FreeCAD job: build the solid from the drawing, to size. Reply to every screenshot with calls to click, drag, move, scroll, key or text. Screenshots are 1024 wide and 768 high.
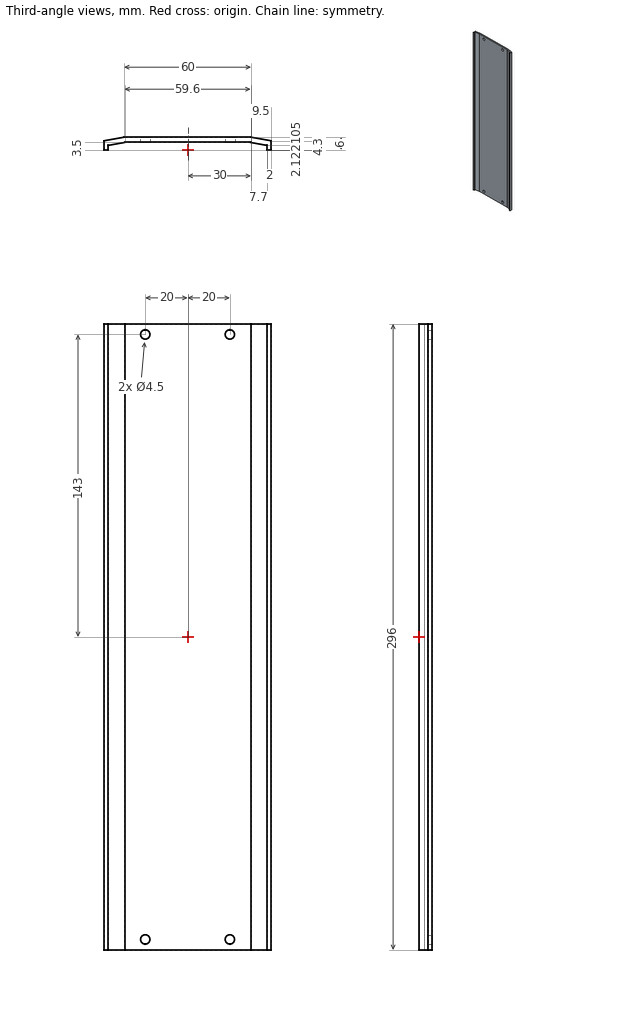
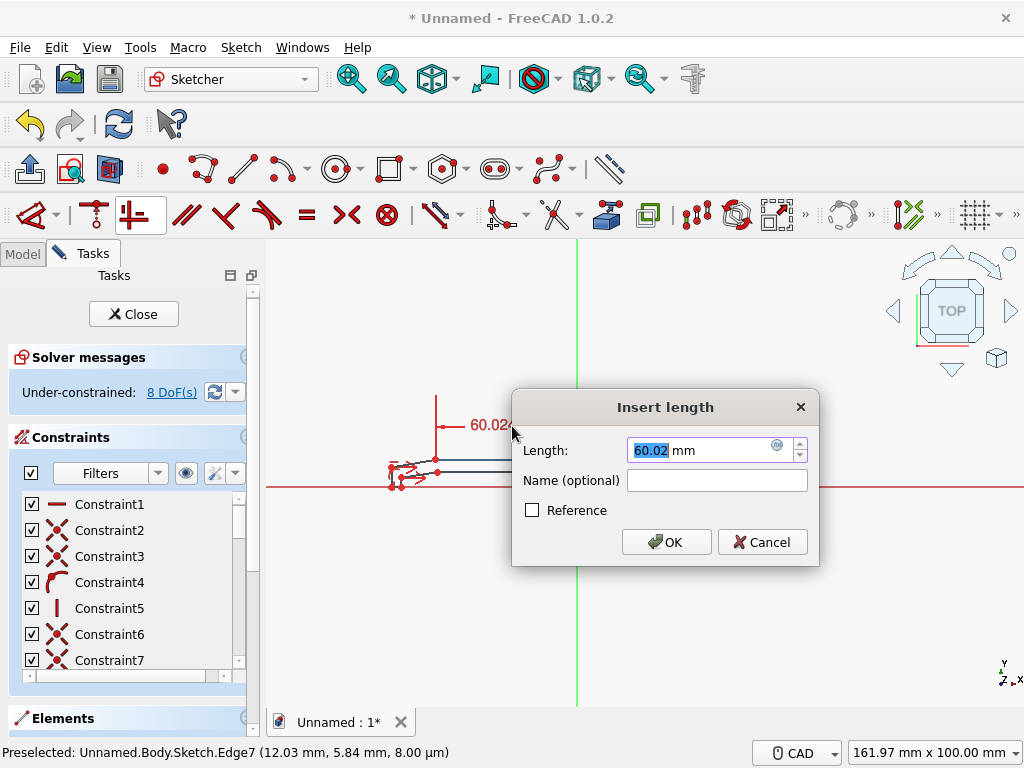
text(60)
key(Return)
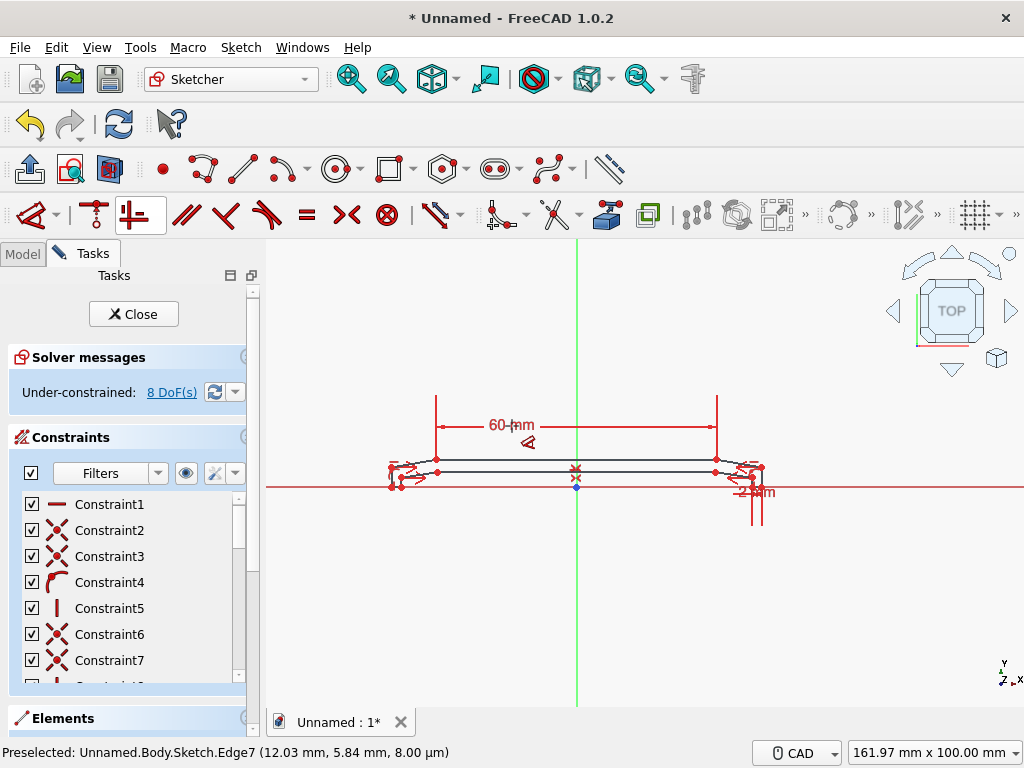
scroll(717, 460, up, 2)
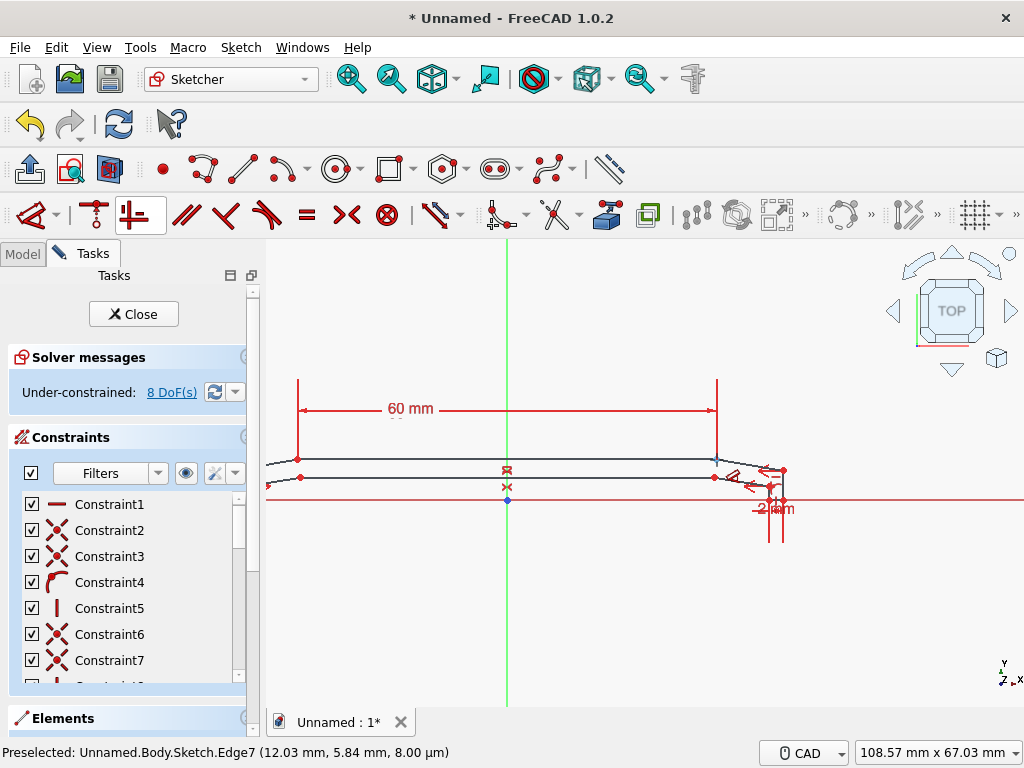
click(717, 459)
click(799, 480)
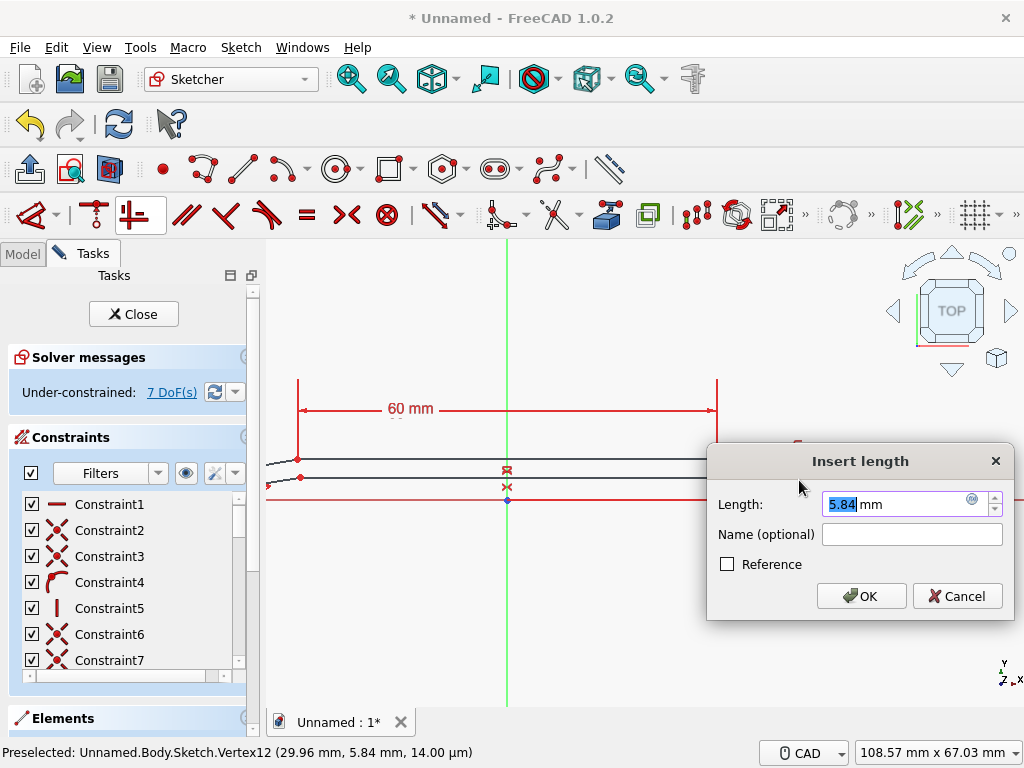
text(6)
key(Return)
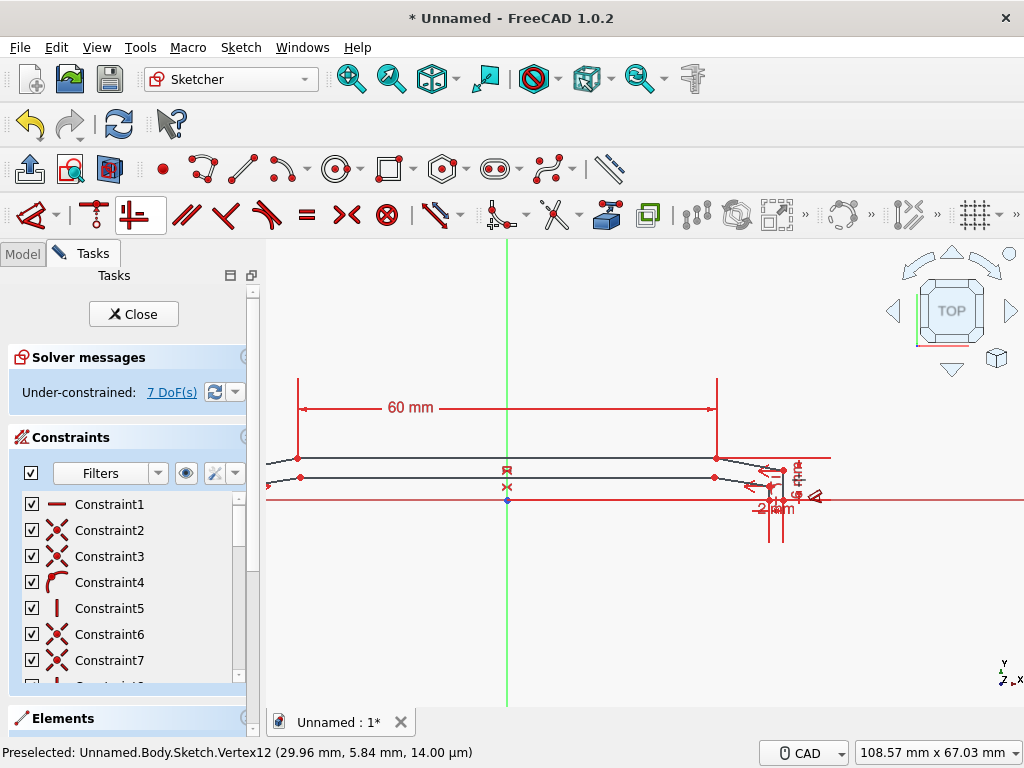
scroll(783, 489, up, 2)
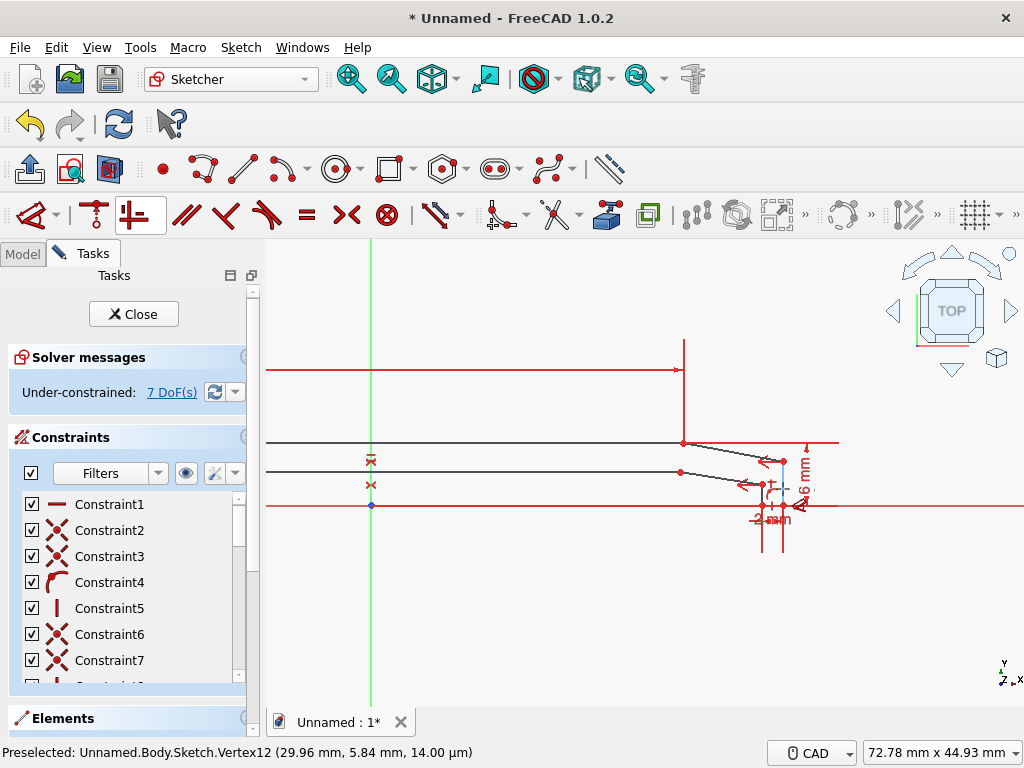
click(783, 488)
click(817, 494)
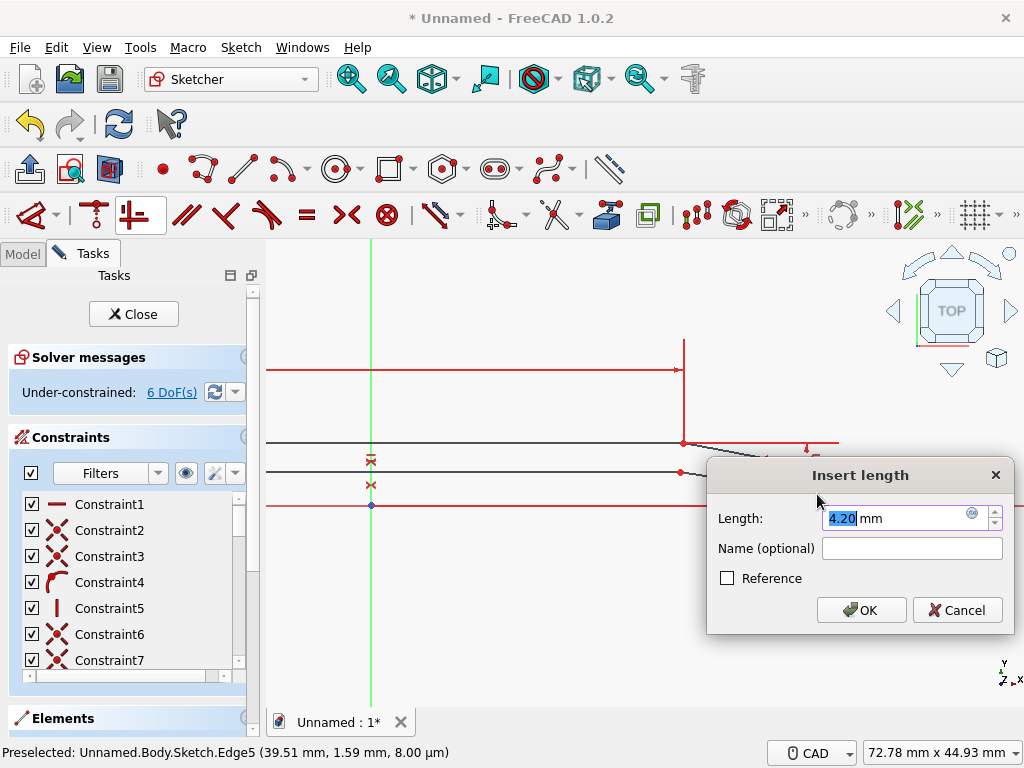
text(4.3)
key(Return)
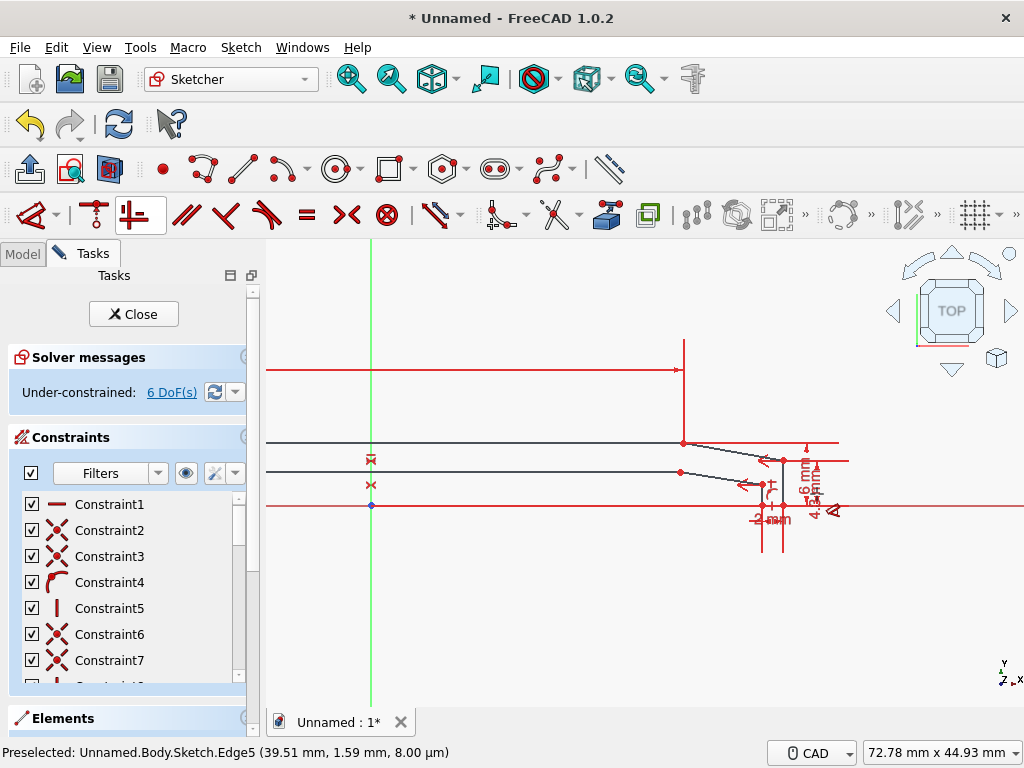
click(684, 443)
click(527, 540)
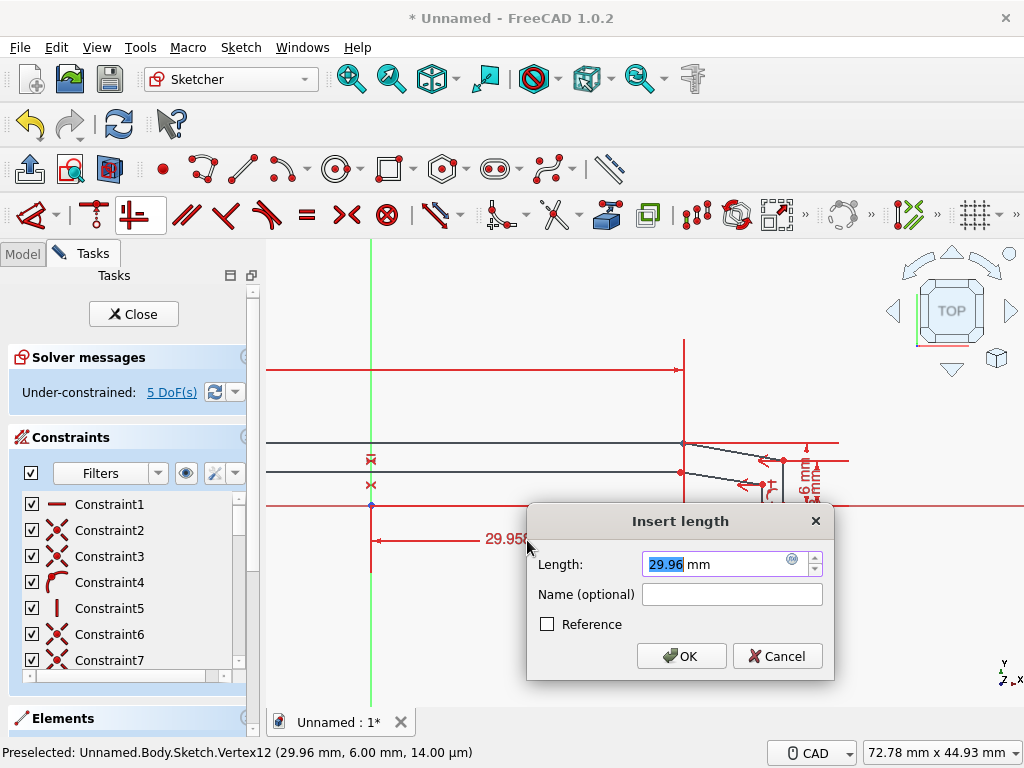
text(30)
key(Return)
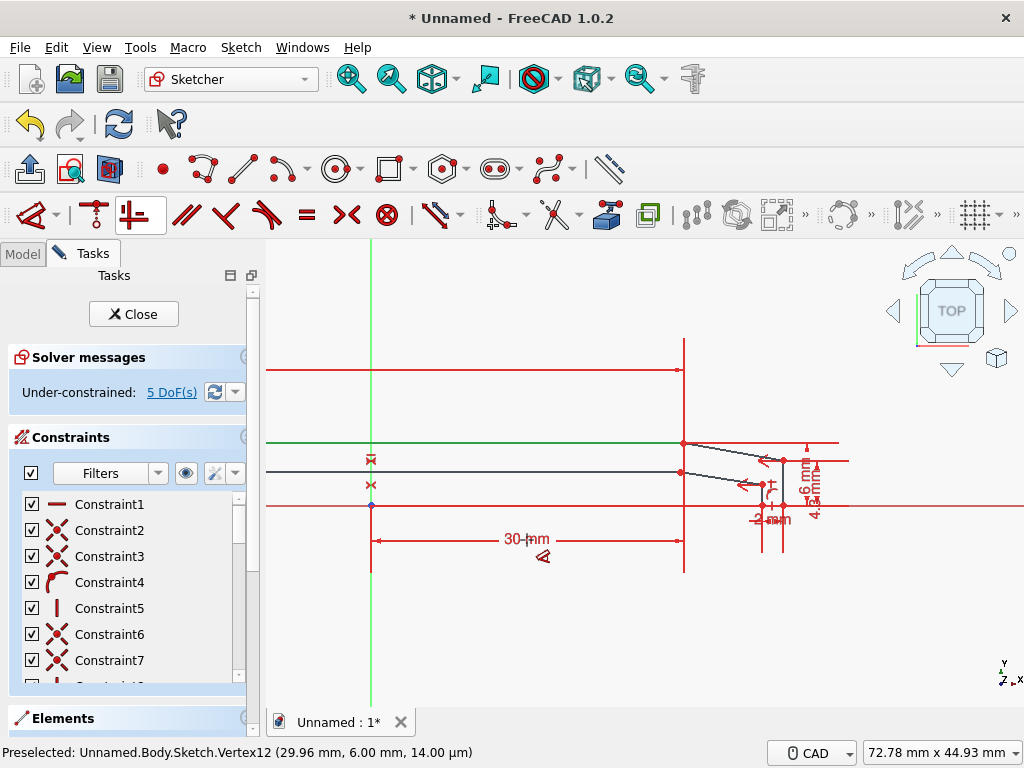
click(495, 472)
click(487, 414)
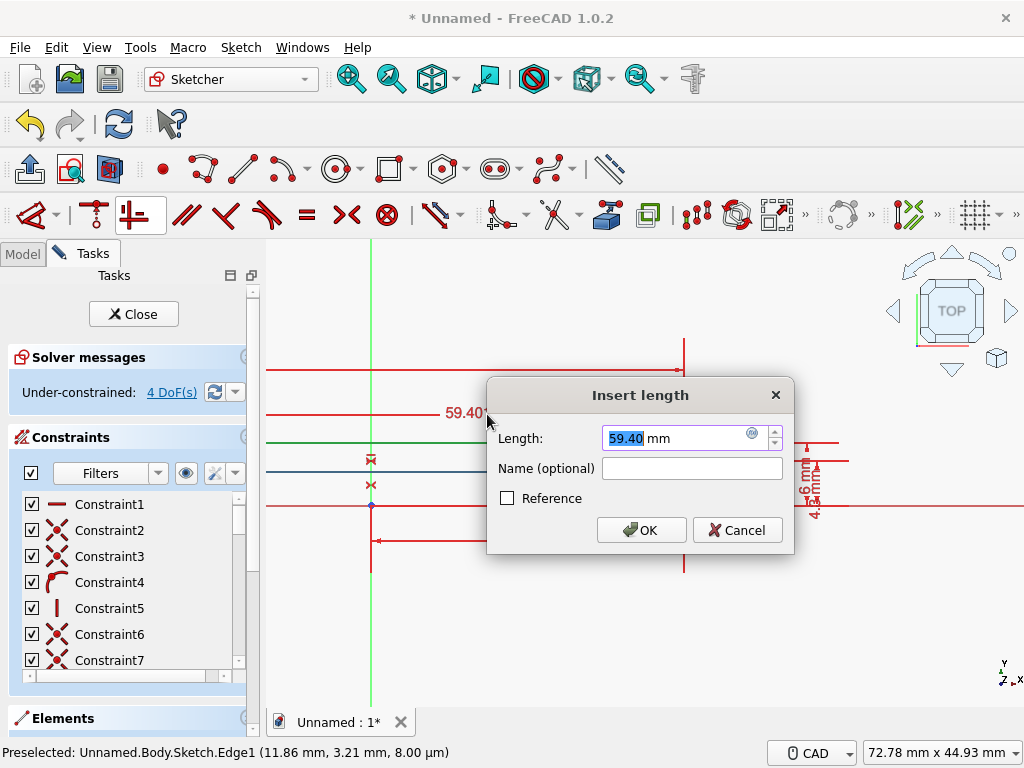
text(59.6)
key(Return)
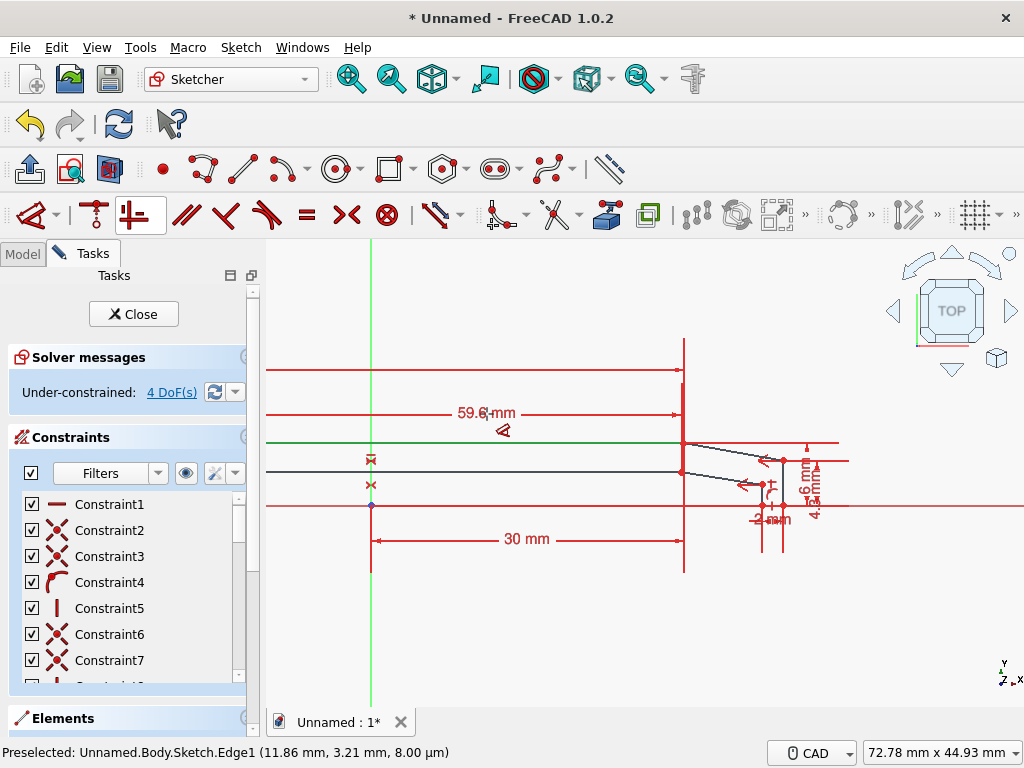
scroll(744, 472, down, 4)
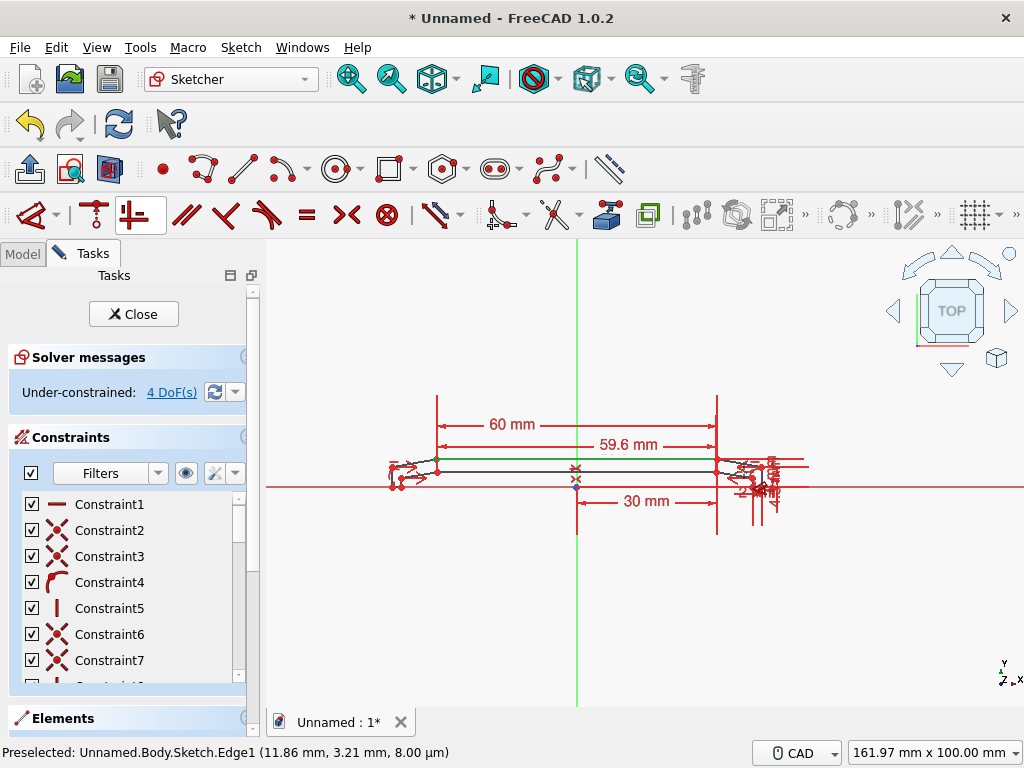
scroll(437, 472, up, 5)